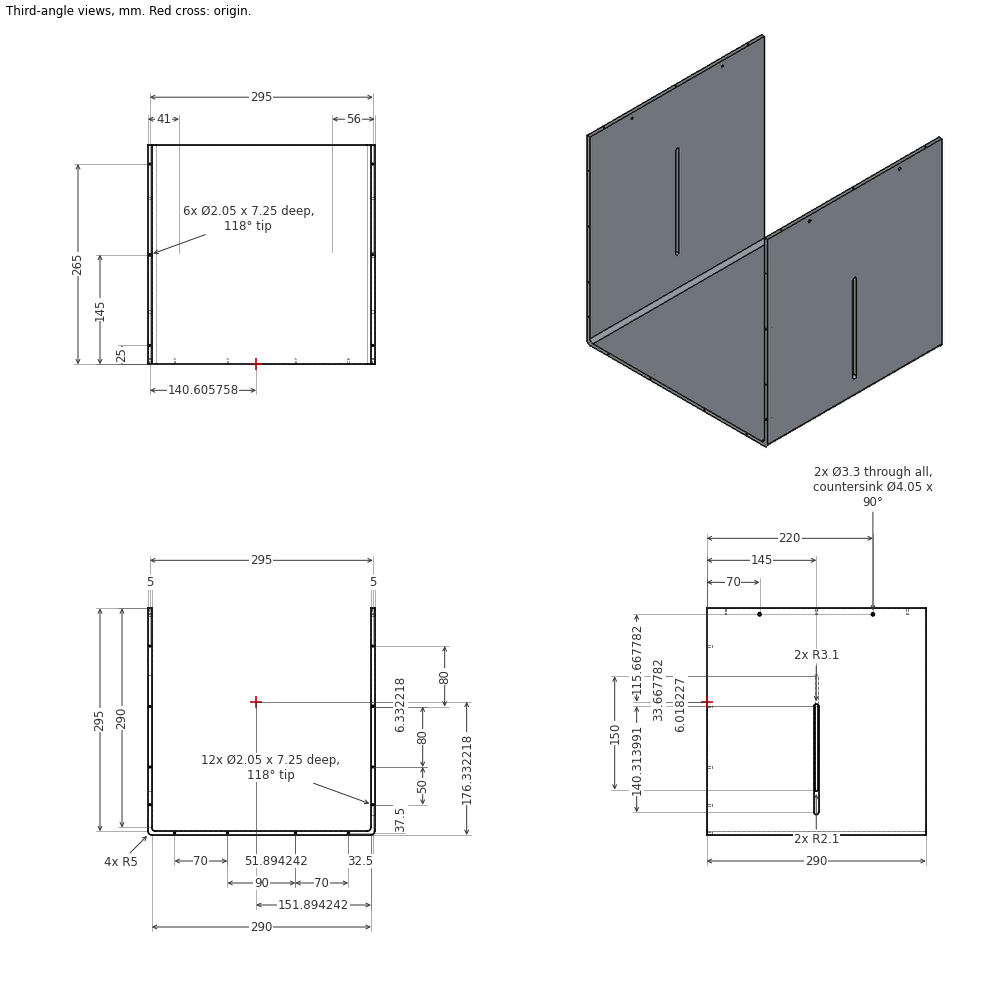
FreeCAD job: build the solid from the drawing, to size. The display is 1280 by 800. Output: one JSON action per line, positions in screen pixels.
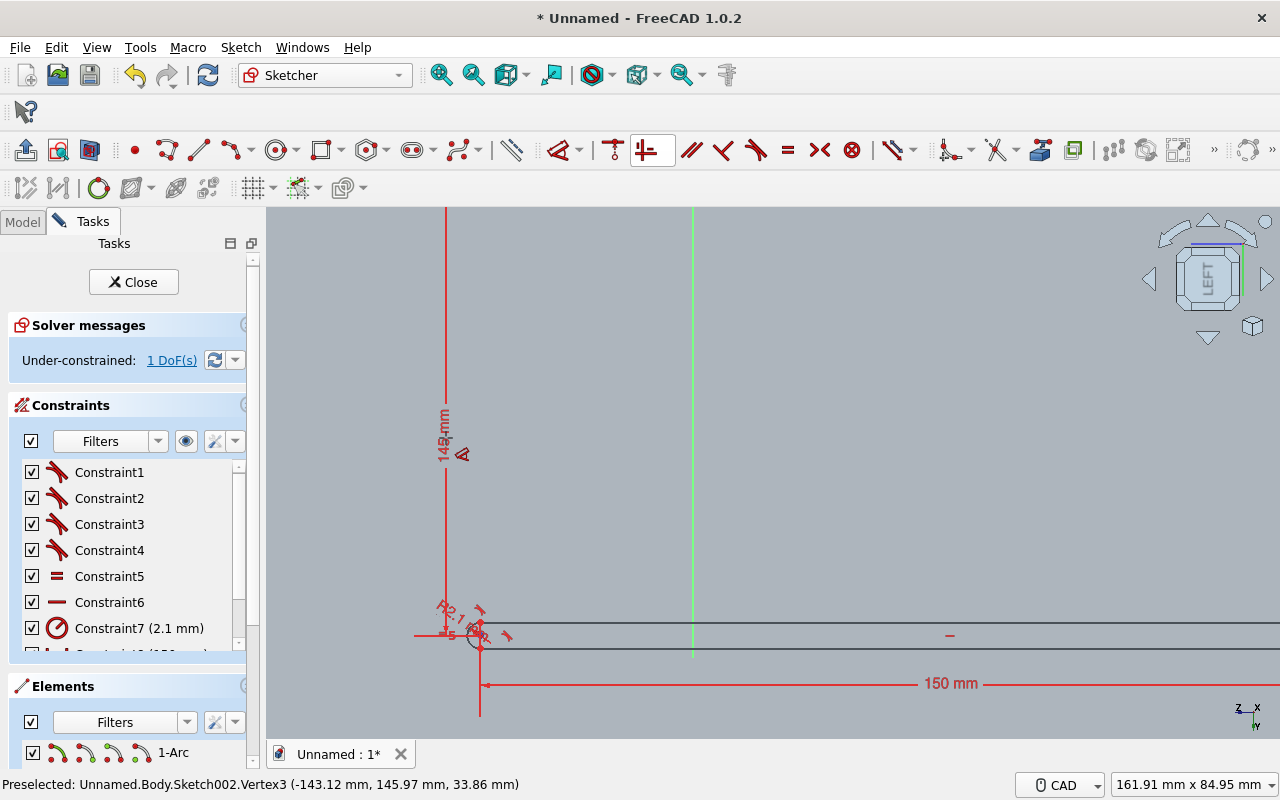
{"action": "left_click", "coordinate": [480, 623]}
{"action": "left_click", "coordinate": [587, 681]}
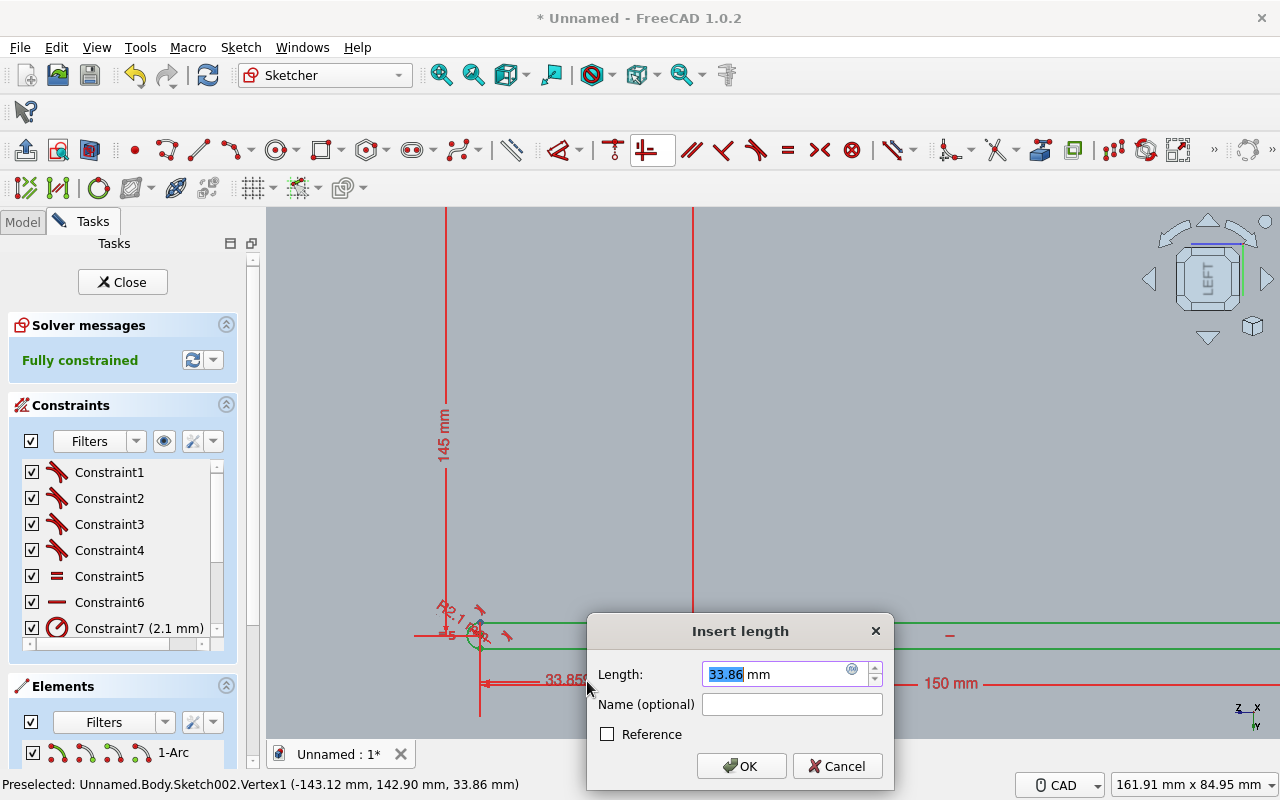
{"action": "type", "text": "33.667782"}
{"action": "key", "text": "Return"}
{"action": "key", "text": "Escape"}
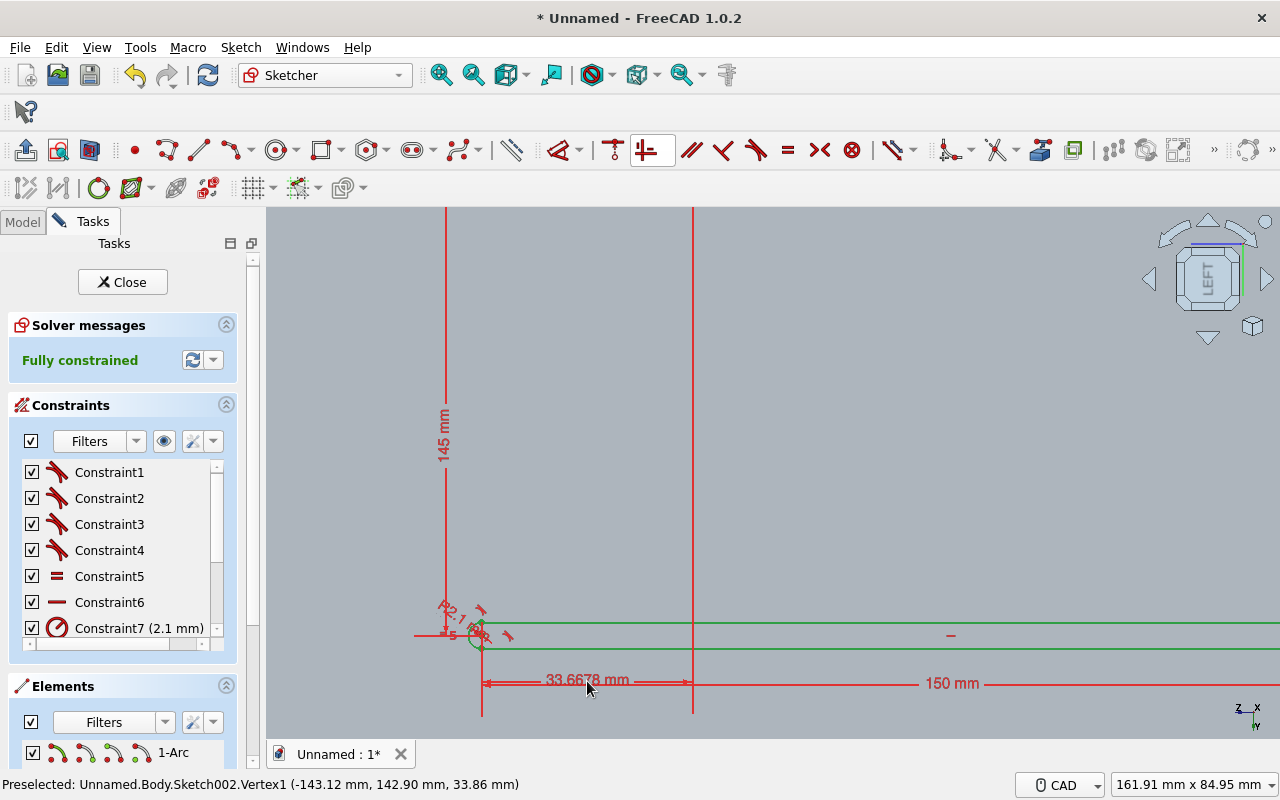
{"action": "left_click", "coordinate": [123, 282]}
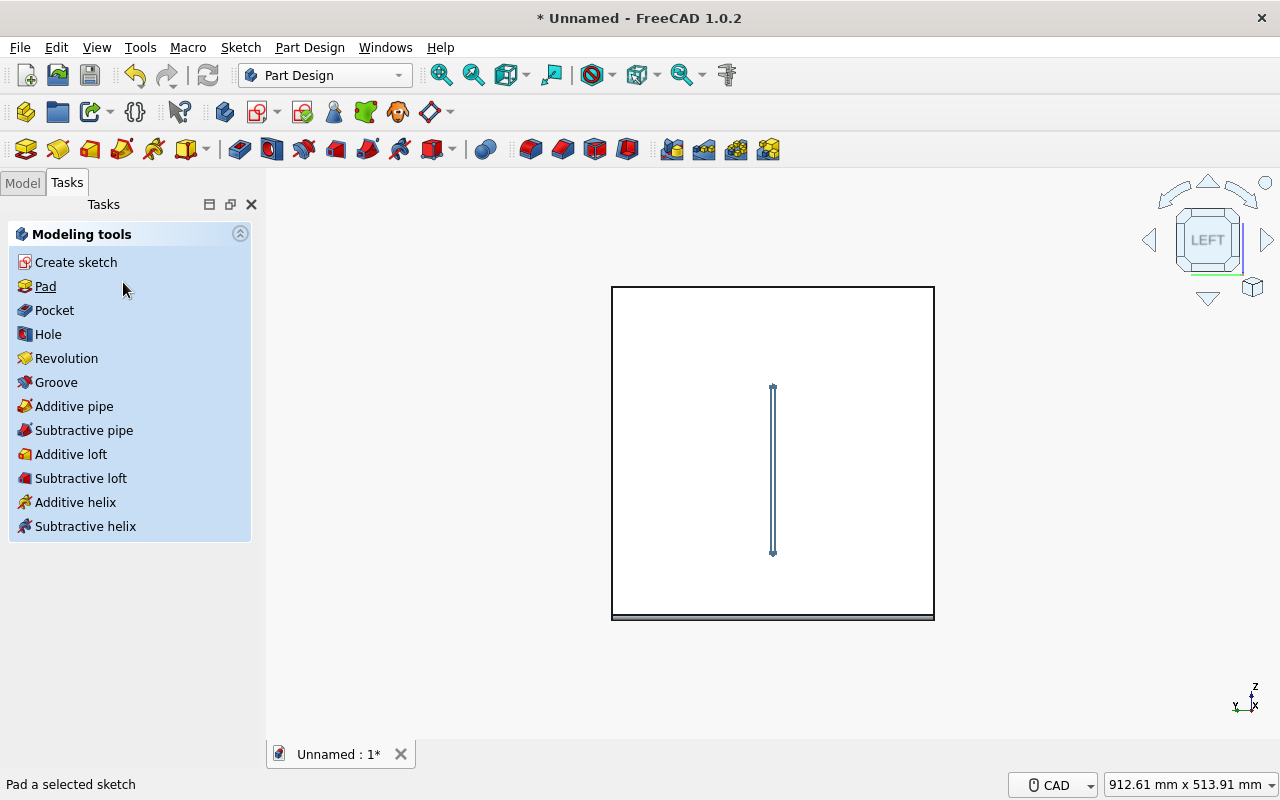
{"action": "left_click", "coordinate": [240, 150]}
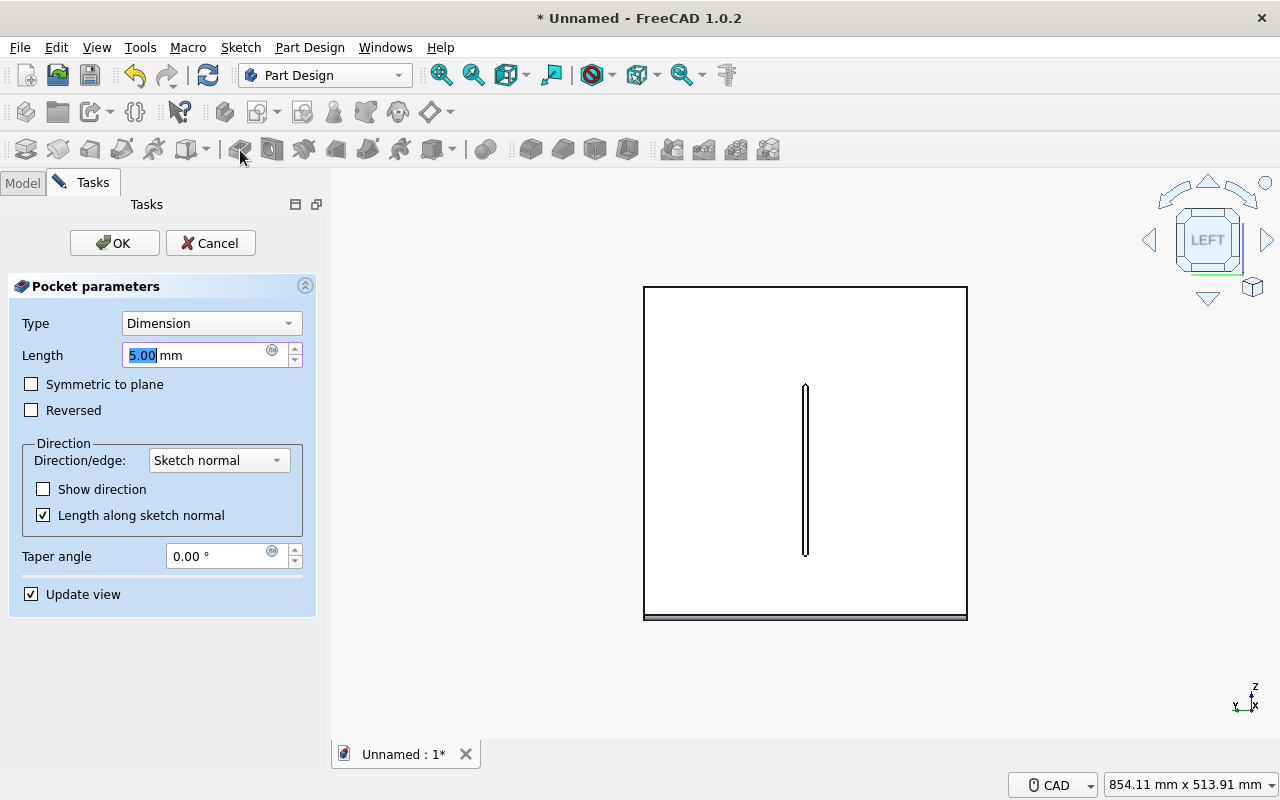
{"action": "type", "text": "41"}
{"action": "key", "text": "Tab"}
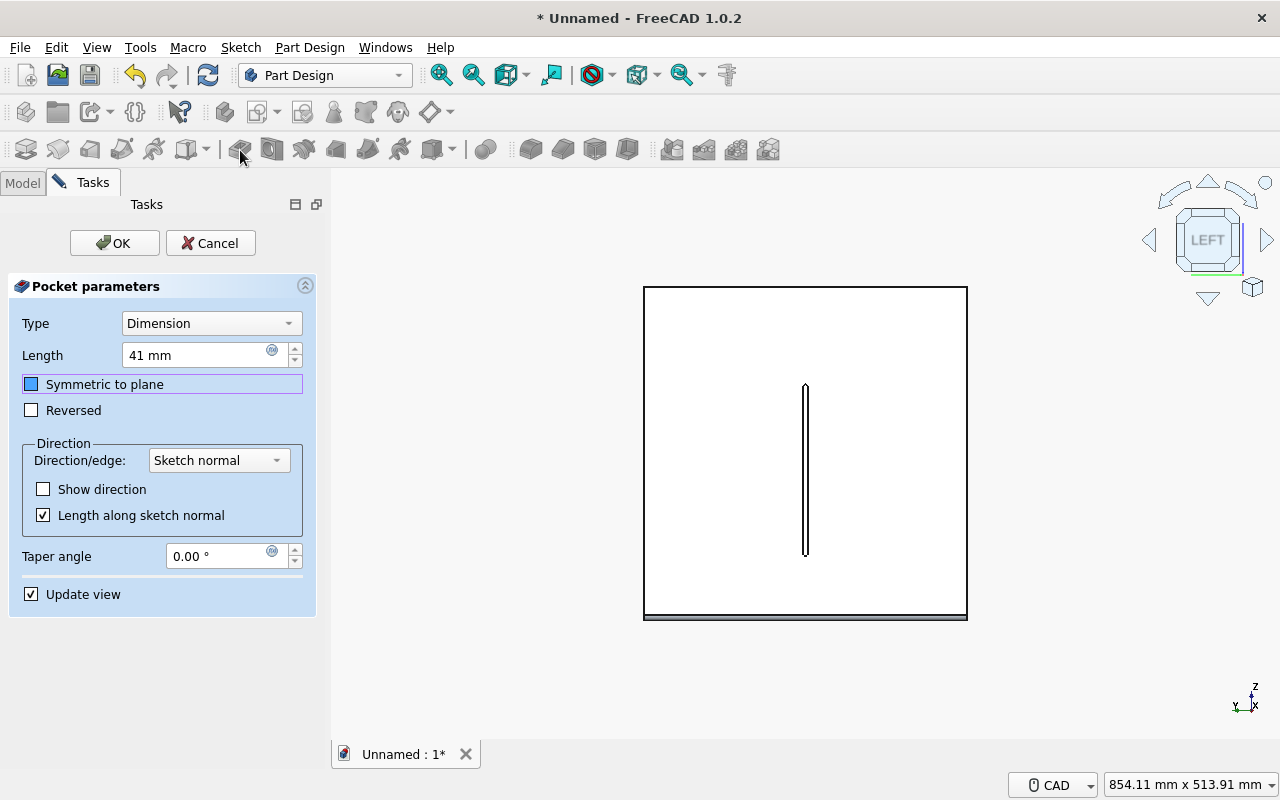
{"action": "left_click", "coordinate": [115, 243]}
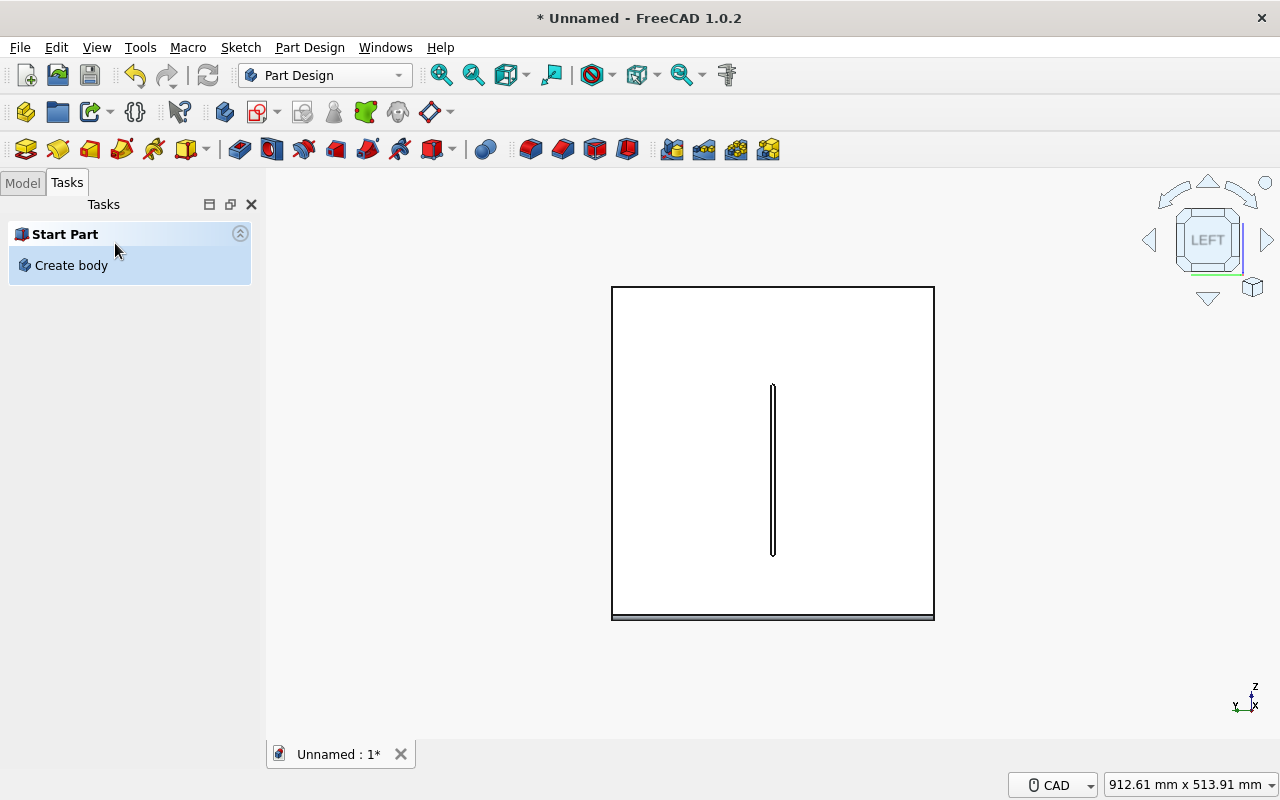
{"action": "key", "text": "0"}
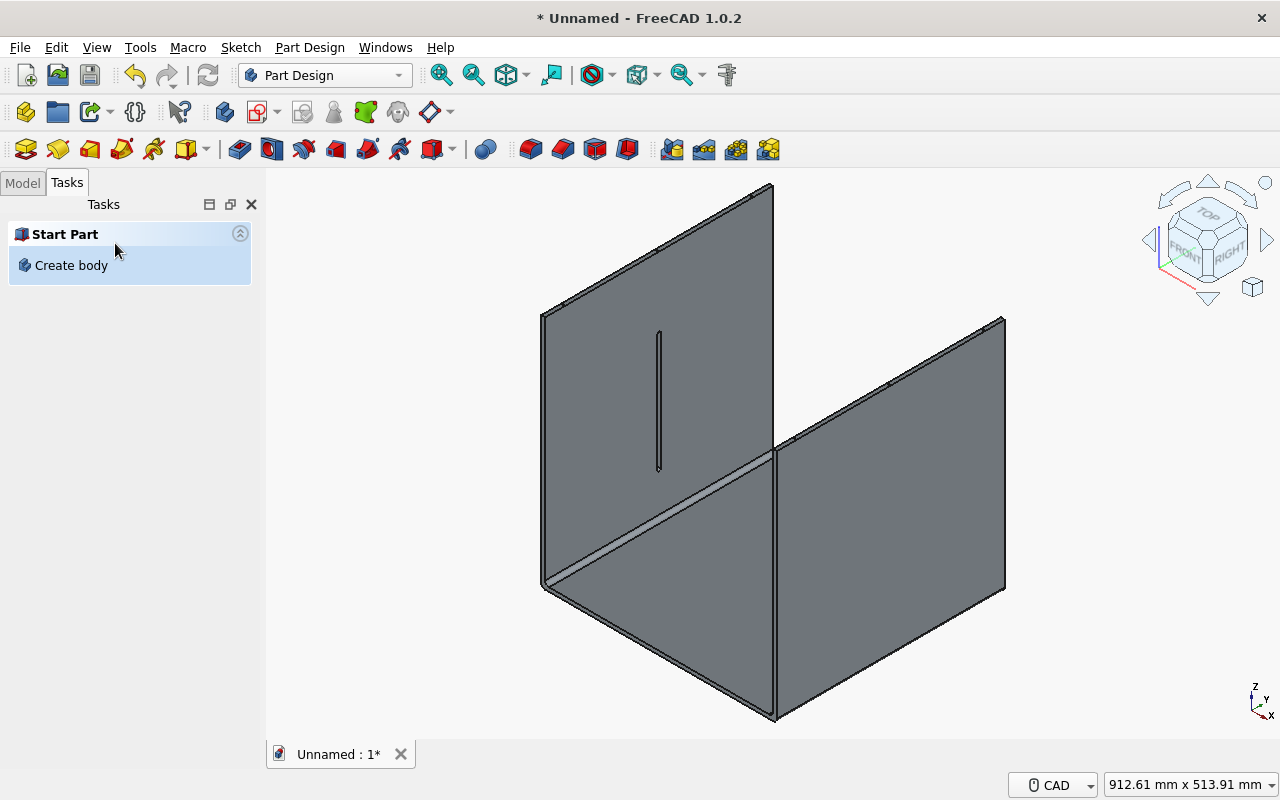
{"action": "left_click", "coordinate": [891, 518]}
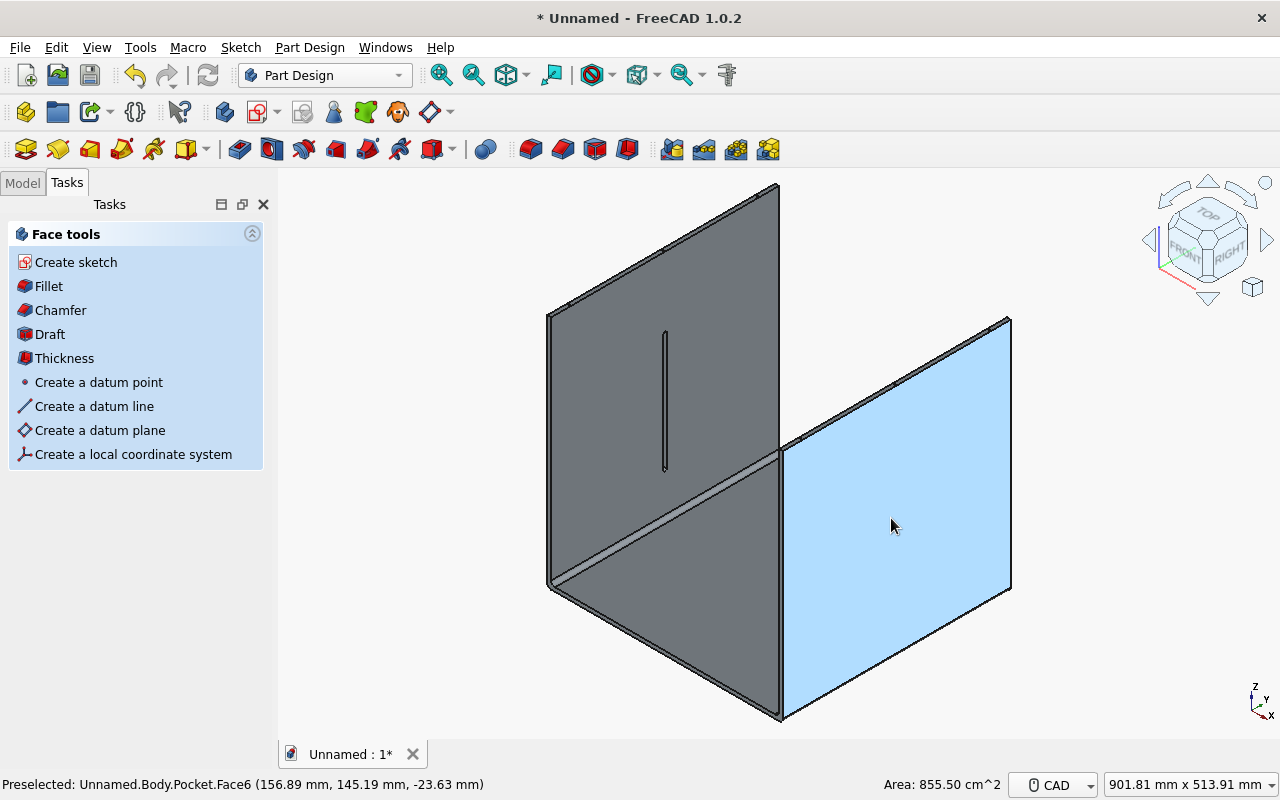
{"action": "left_click", "coordinate": [258, 112]}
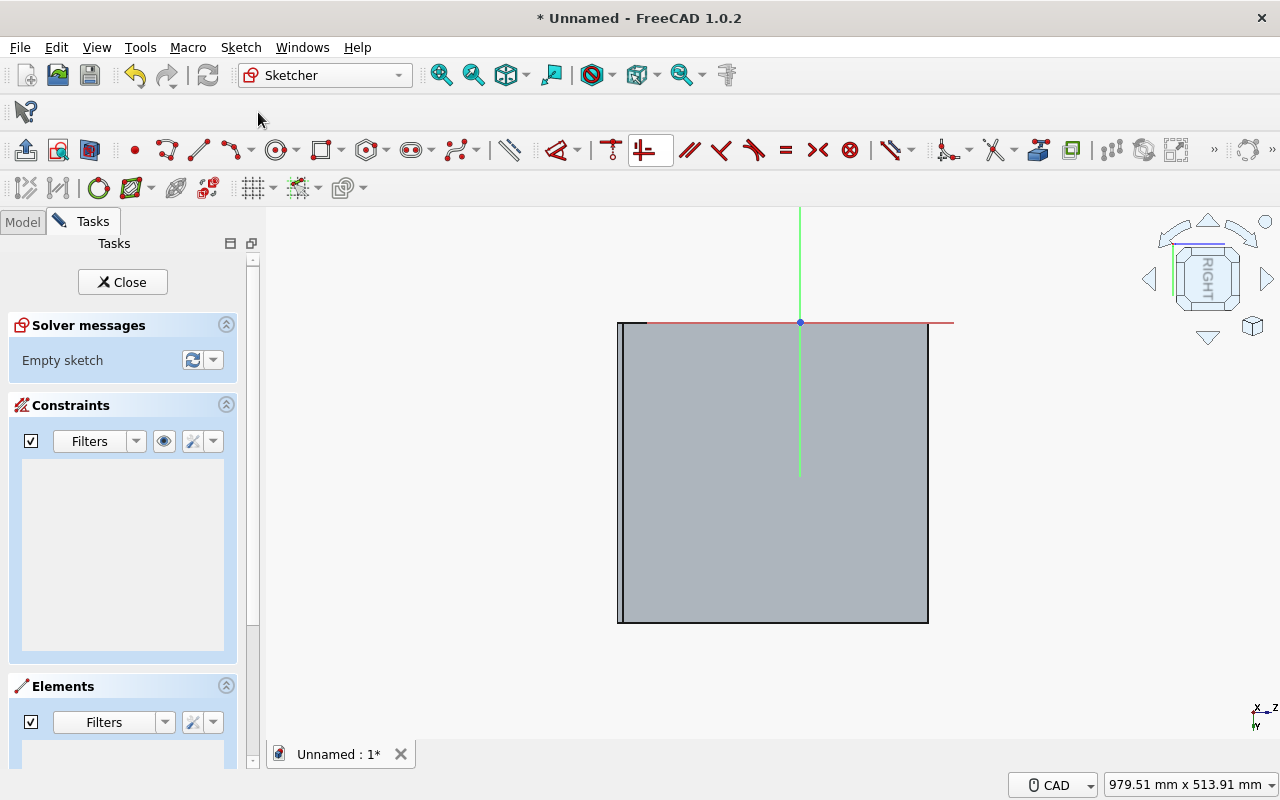
{"action": "scroll", "coordinate": [738, 340], "scroll_direction": "up", "scroll_amount": 4}